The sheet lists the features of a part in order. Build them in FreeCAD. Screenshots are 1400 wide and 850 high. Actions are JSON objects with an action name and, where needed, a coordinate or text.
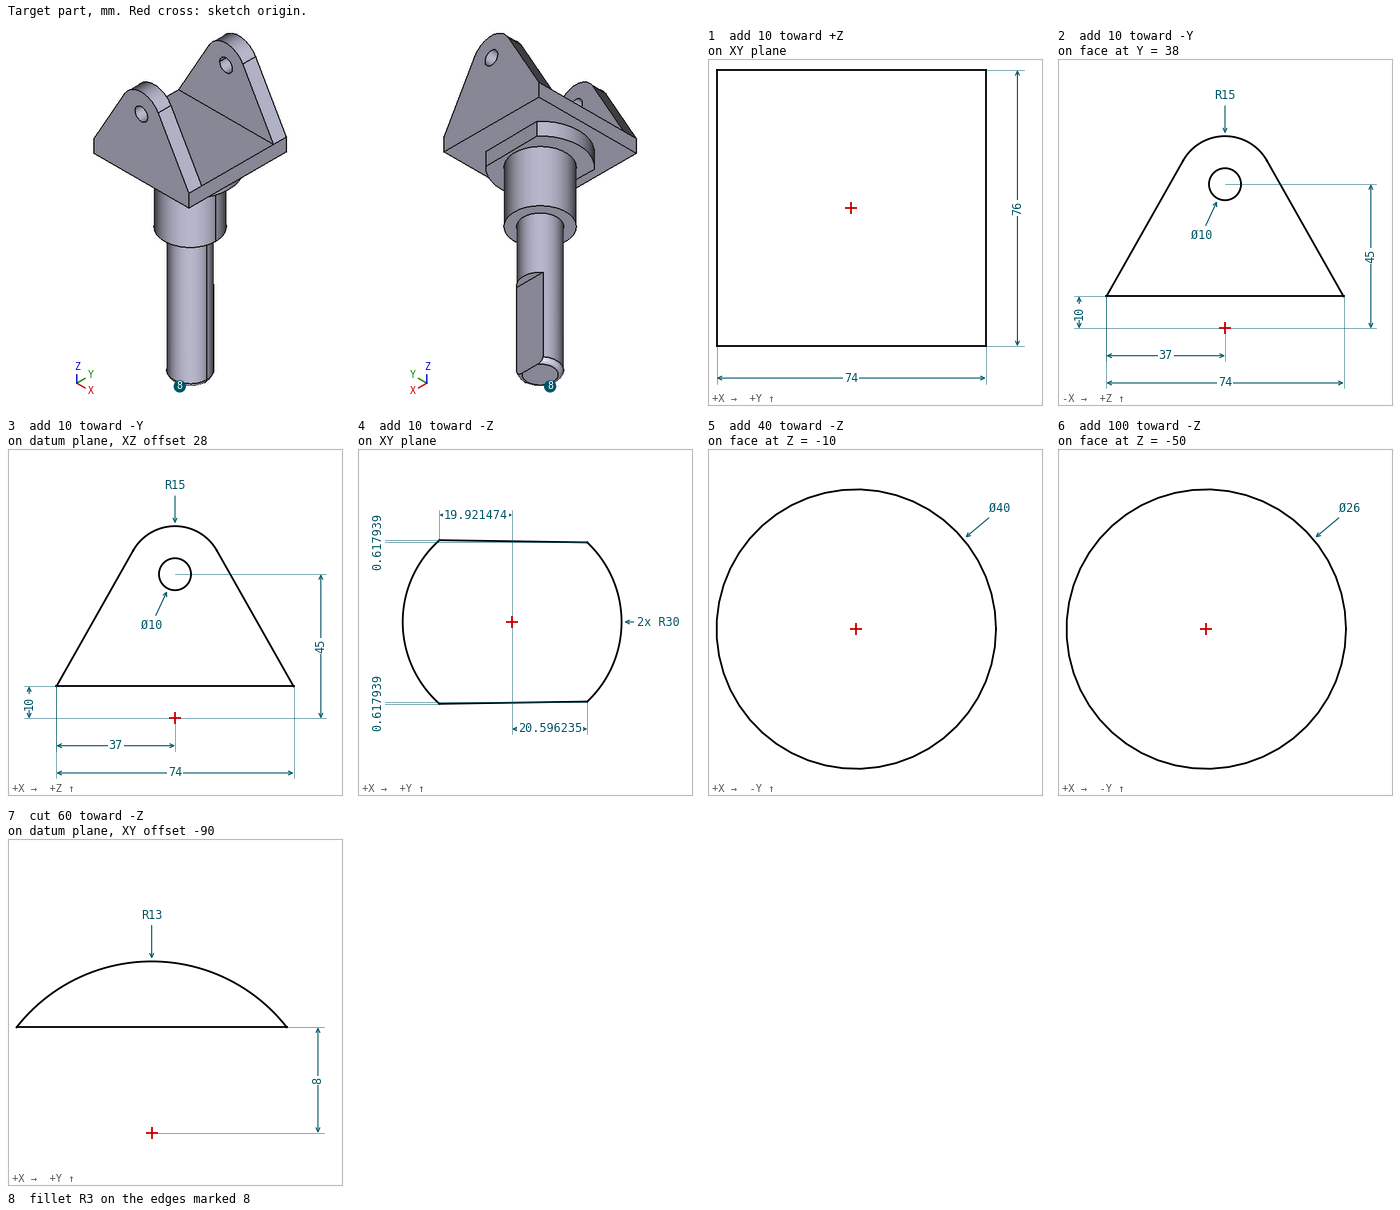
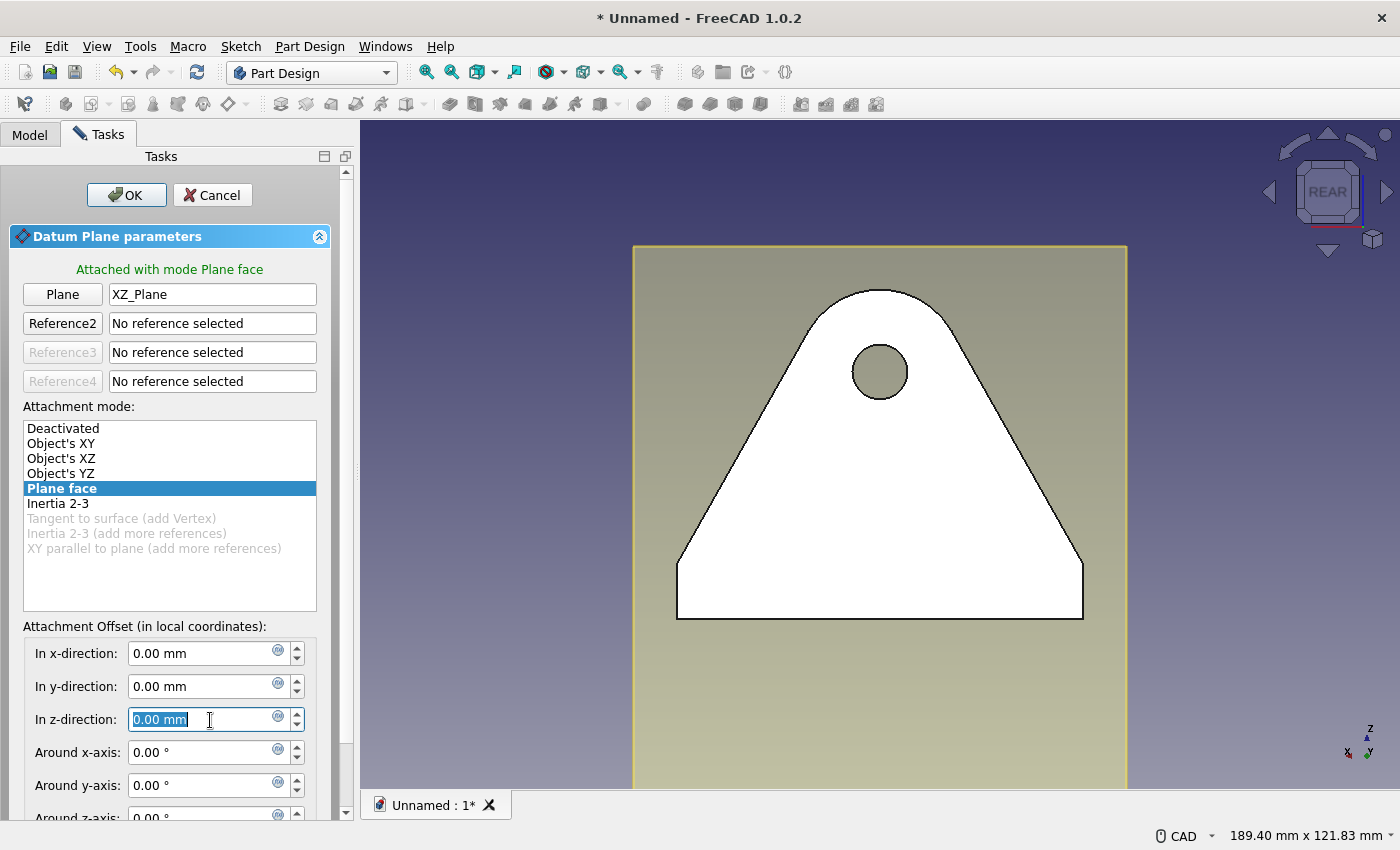
{"action": "type", "text": "28"}
{"action": "key", "text": "Tab"}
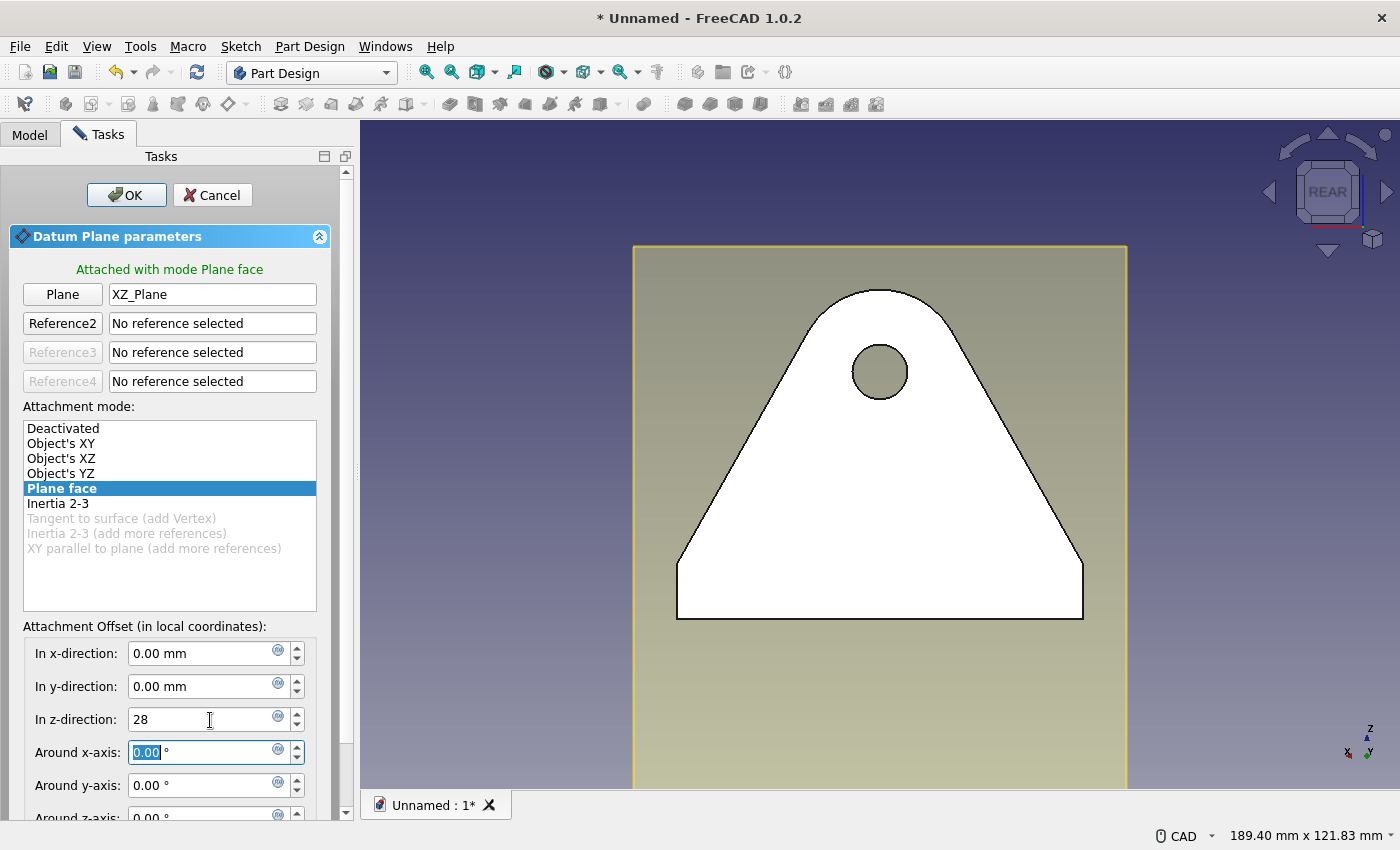
{"action": "left_click", "coordinate": [127, 195]}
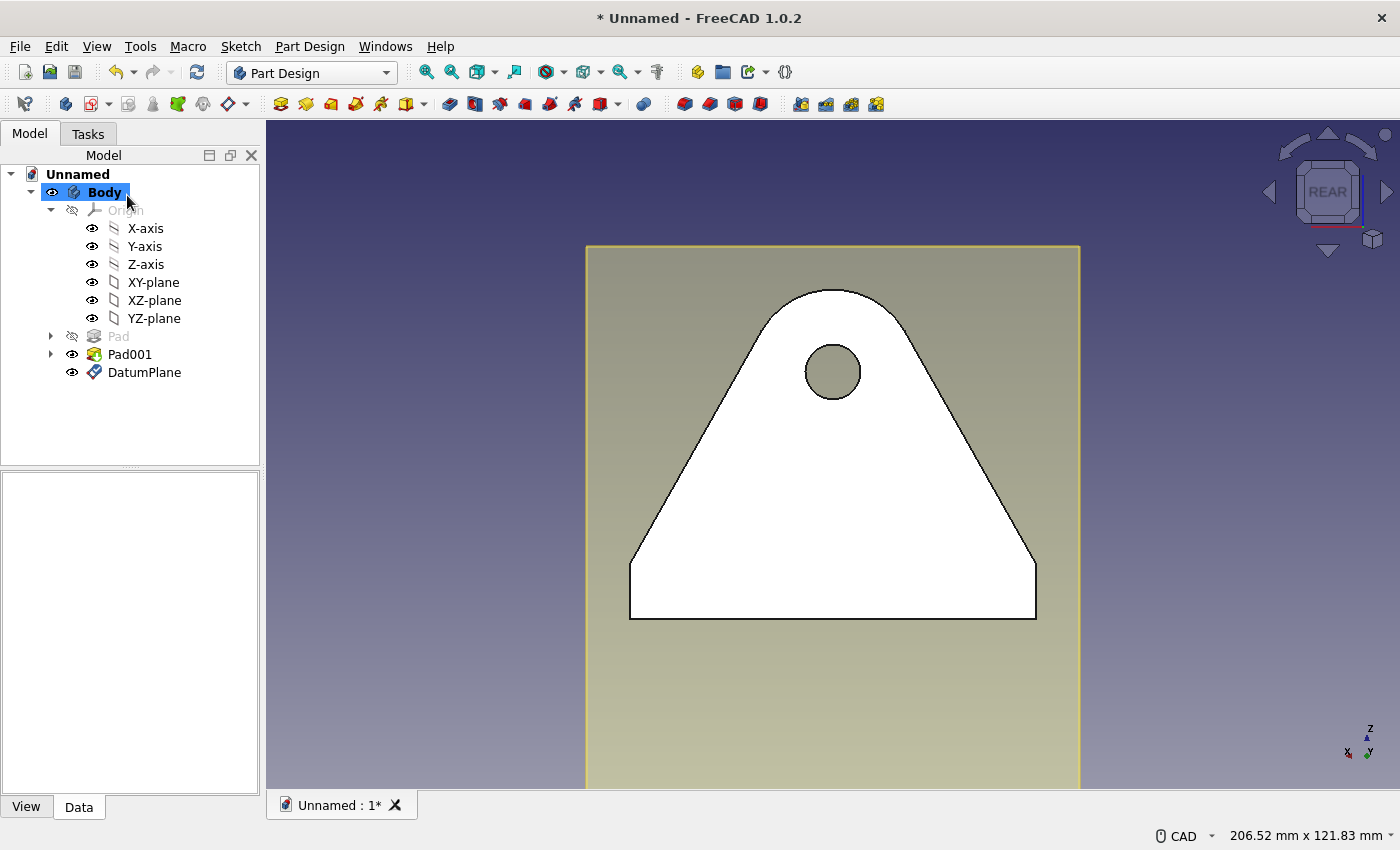
{"action": "left_click", "coordinate": [117, 372]}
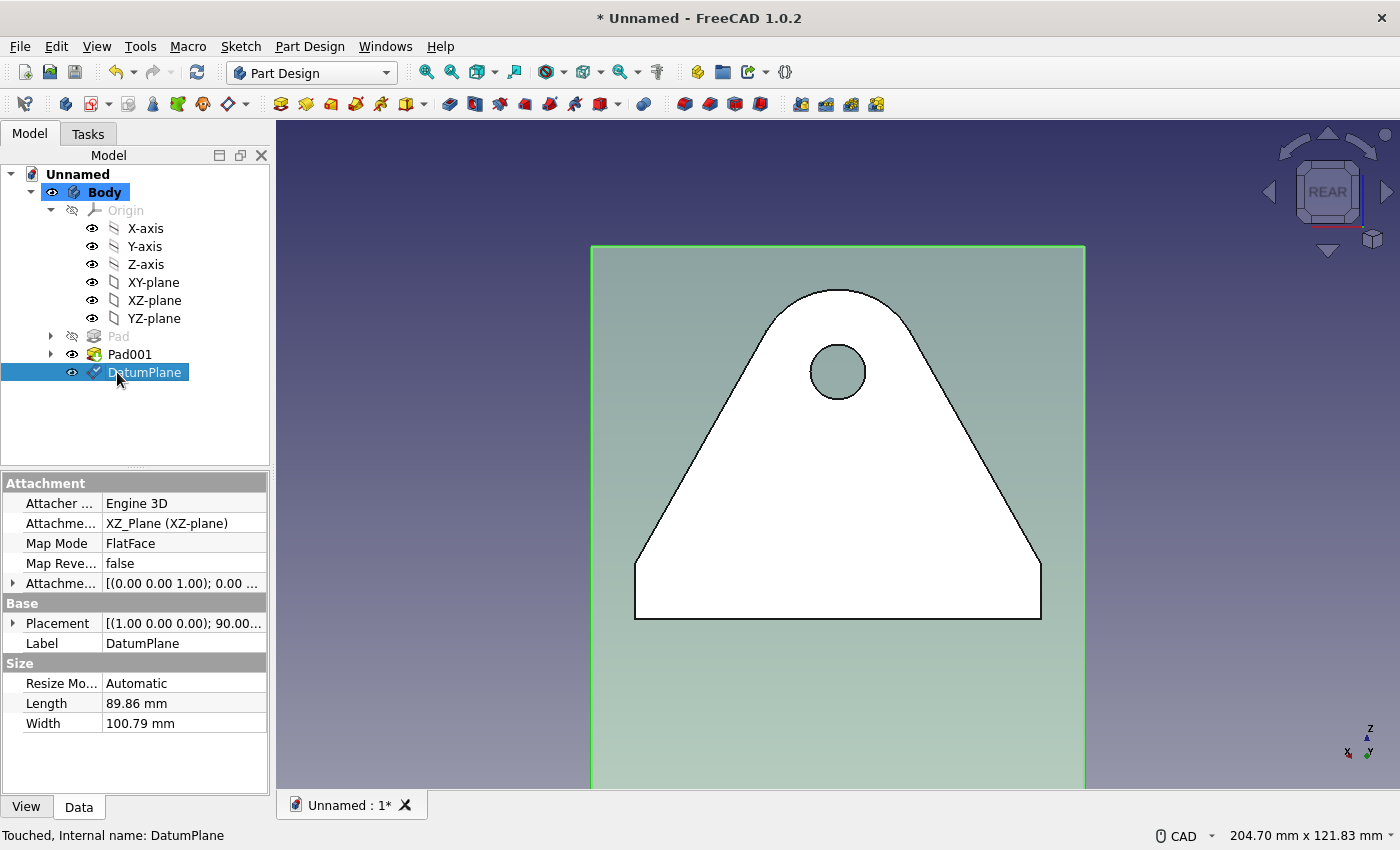
{"action": "left_click", "coordinate": [90, 104]}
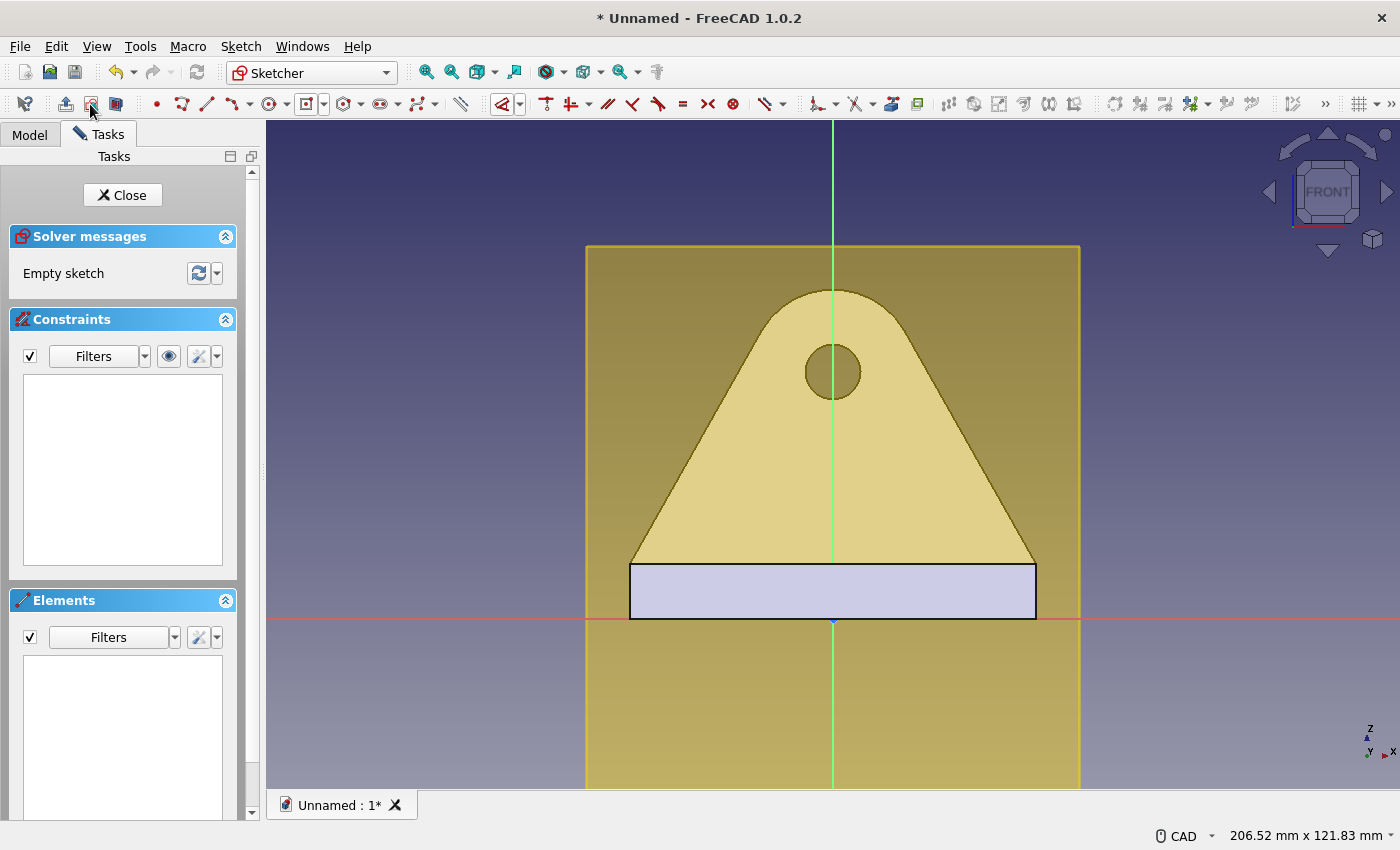
{"action": "key", "text": "q s"}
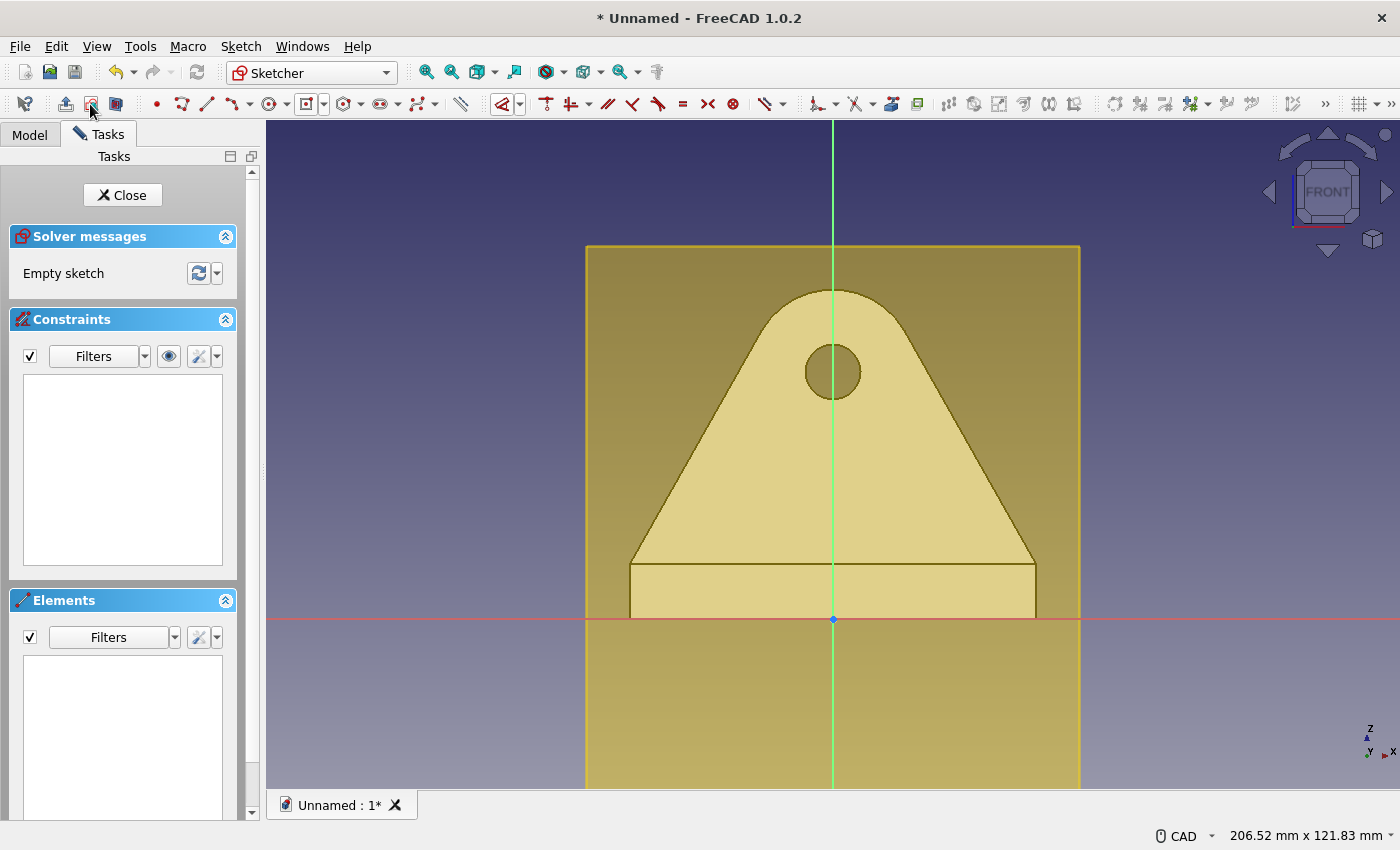
{"action": "left_click", "coordinate": [182, 104]}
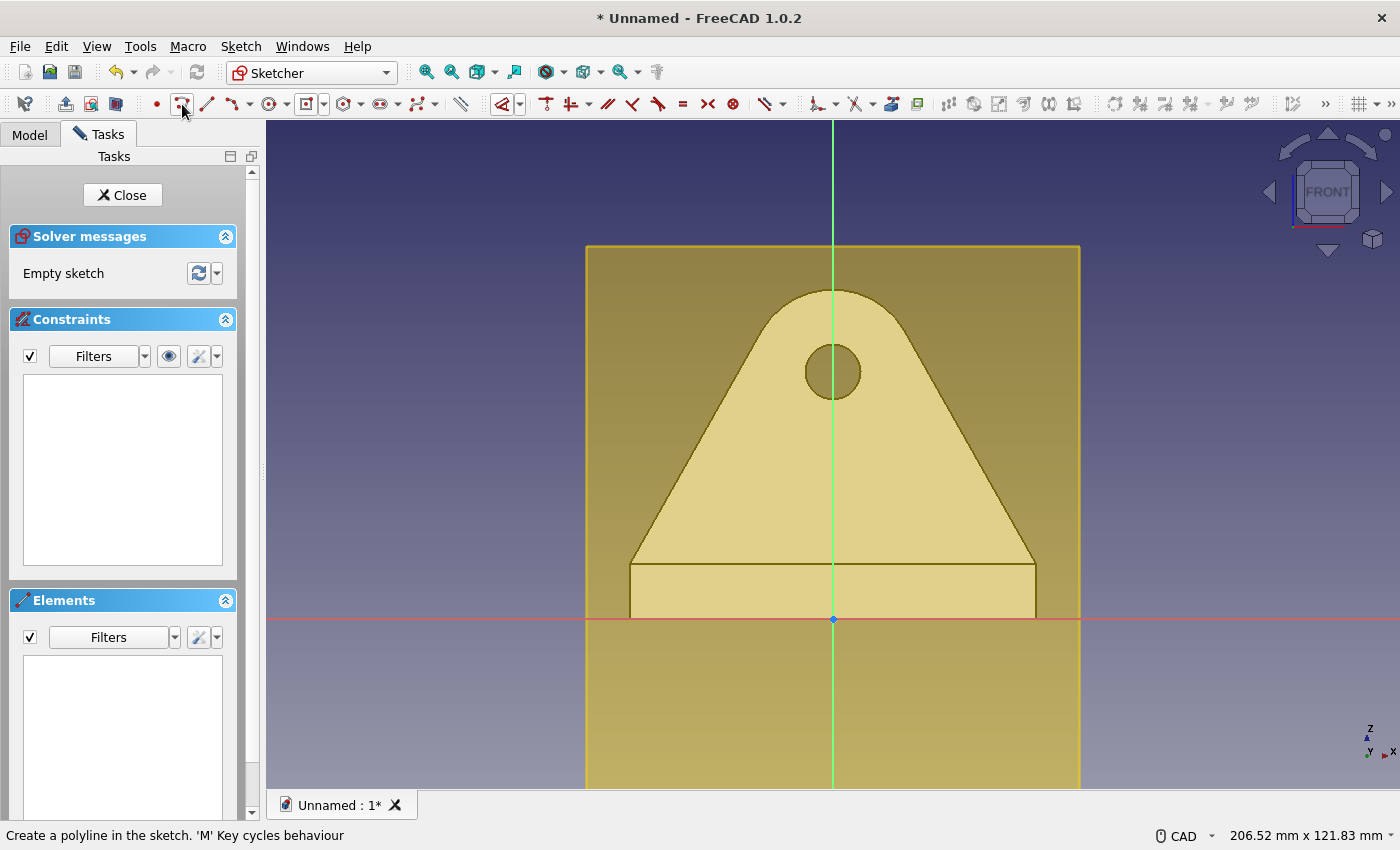
{"action": "left_click", "coordinate": [761, 331]}
{"action": "left_click", "coordinate": [630, 564]}
{"action": "left_click", "coordinate": [1036, 564]}
{"action": "left_click", "coordinate": [905, 331]}
{"action": "right_click", "coordinate": [905, 331]}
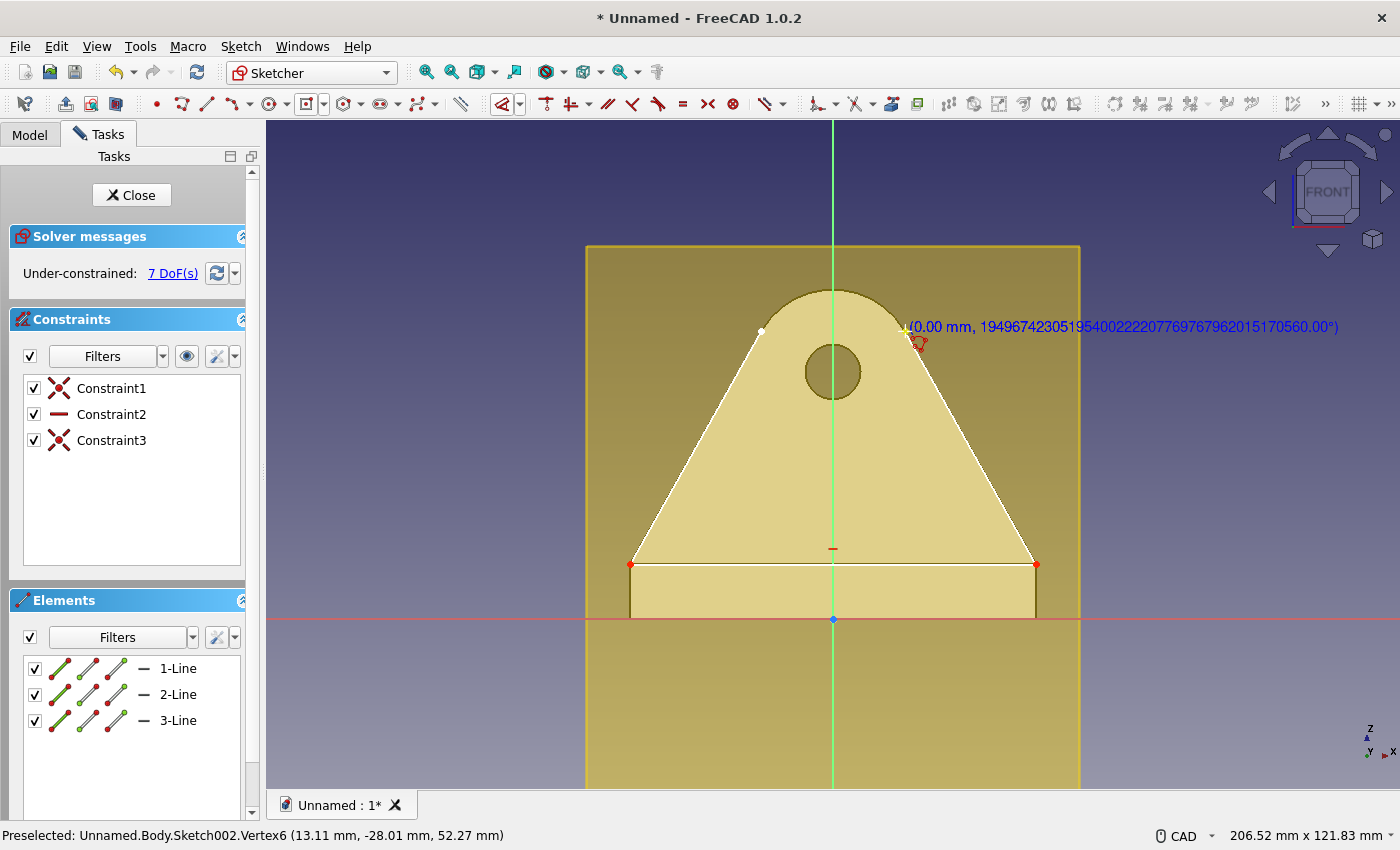
{"action": "left_click", "coordinate": [232, 104]}